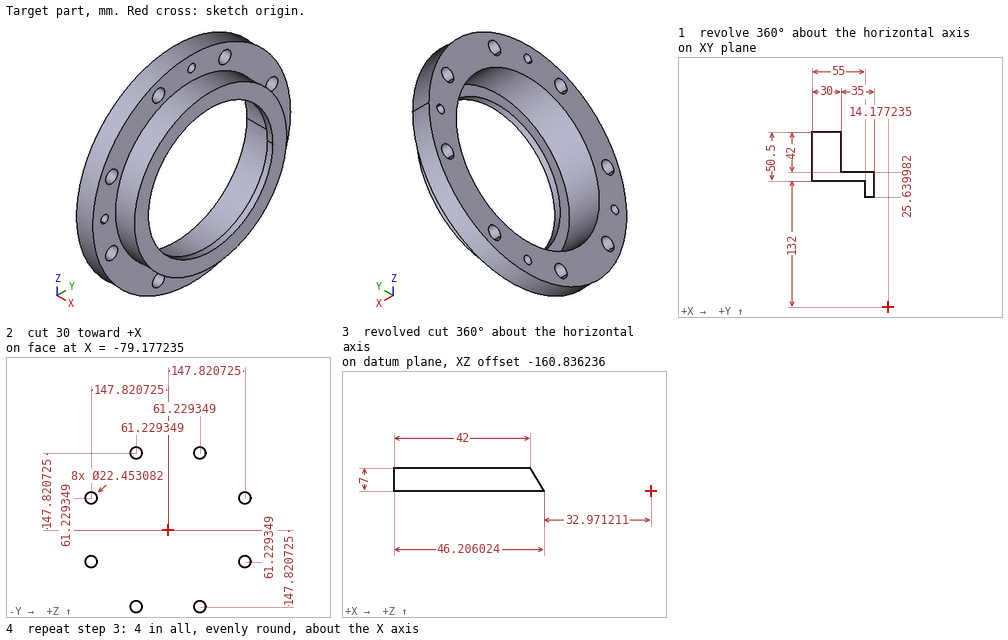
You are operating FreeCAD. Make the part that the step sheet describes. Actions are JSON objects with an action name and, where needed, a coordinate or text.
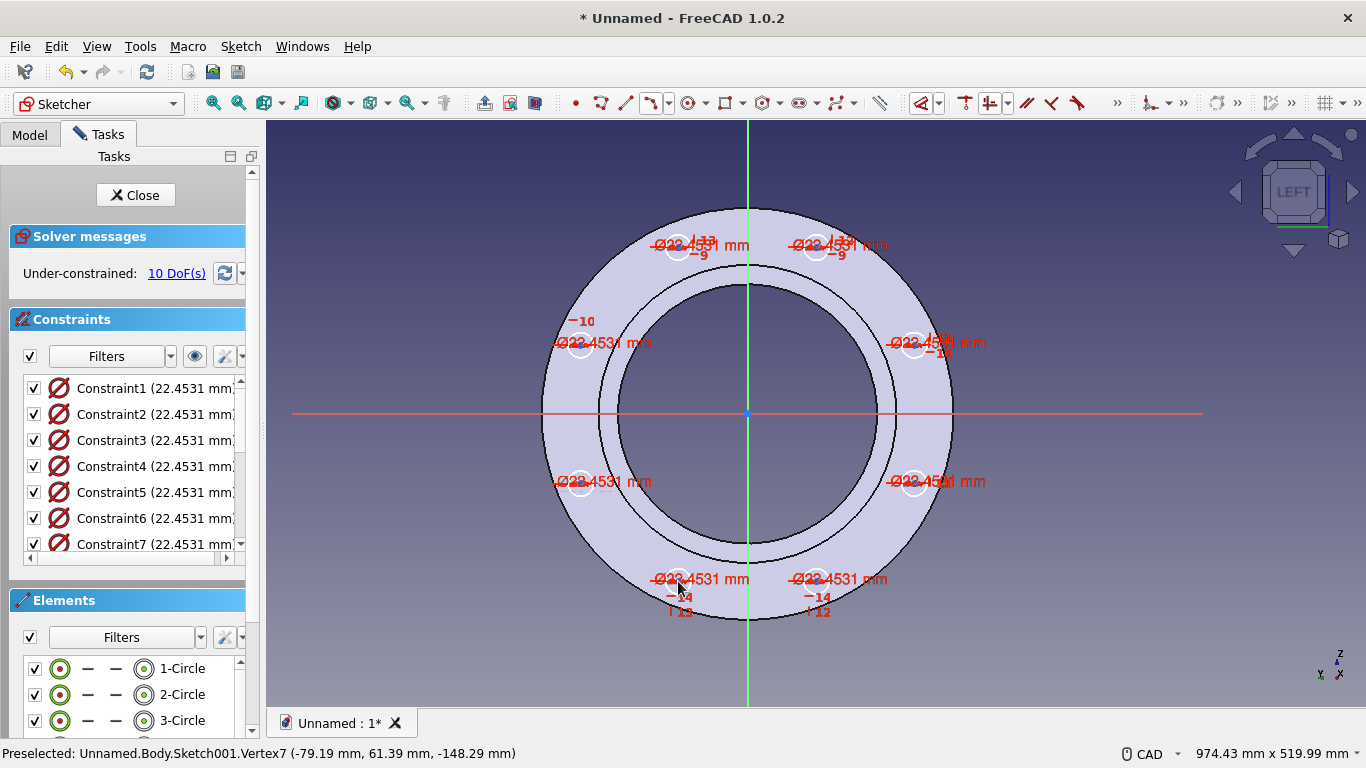
{"action": "left_click", "coordinate": [581, 345]}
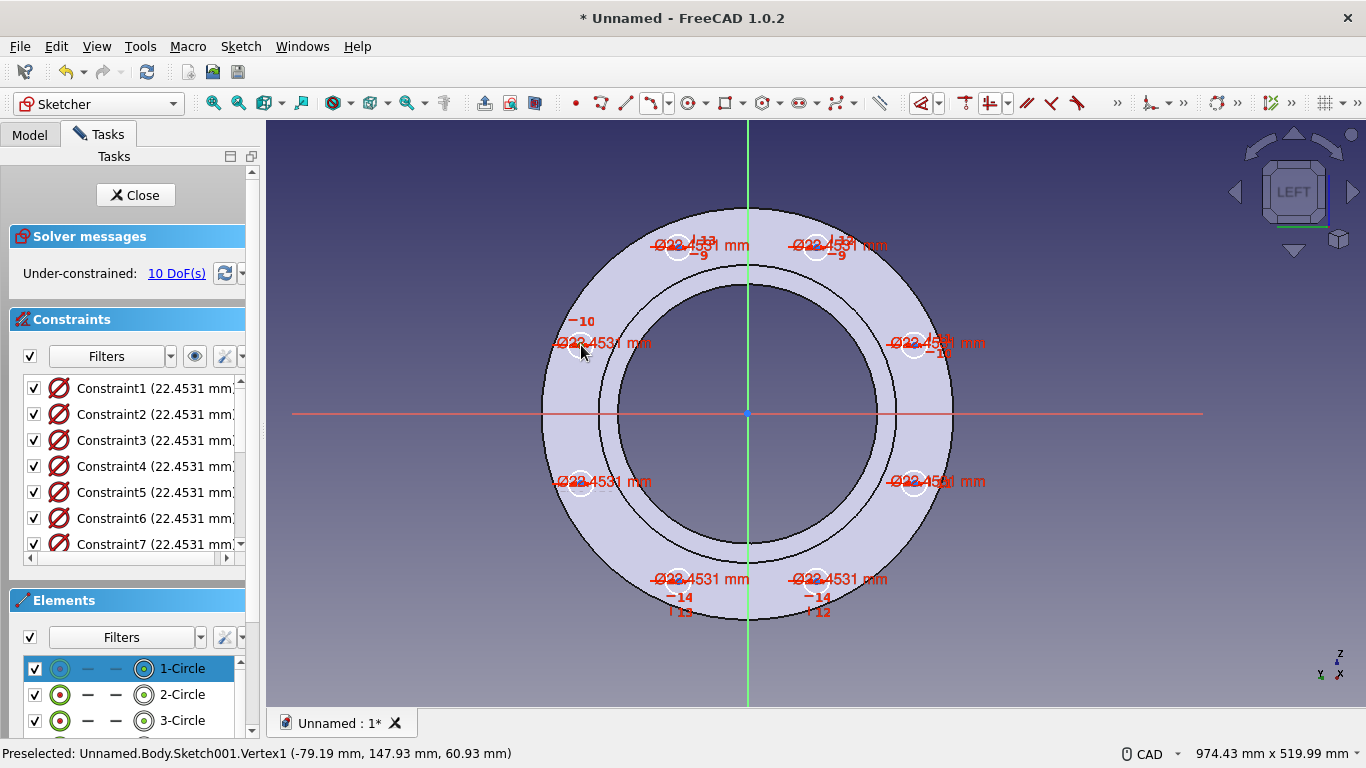
{"action": "left_click", "coordinate": [581, 484]}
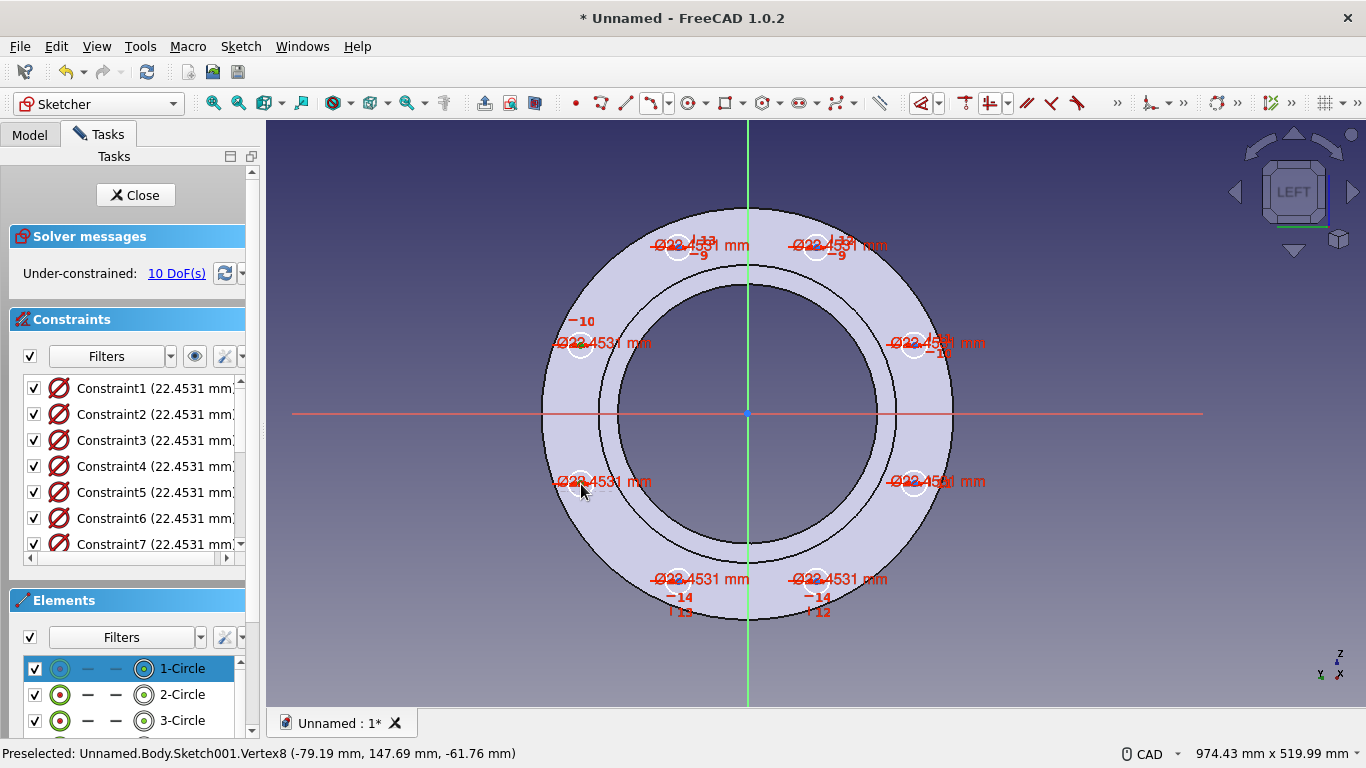
{"action": "left_click", "coordinate": [1008, 104]}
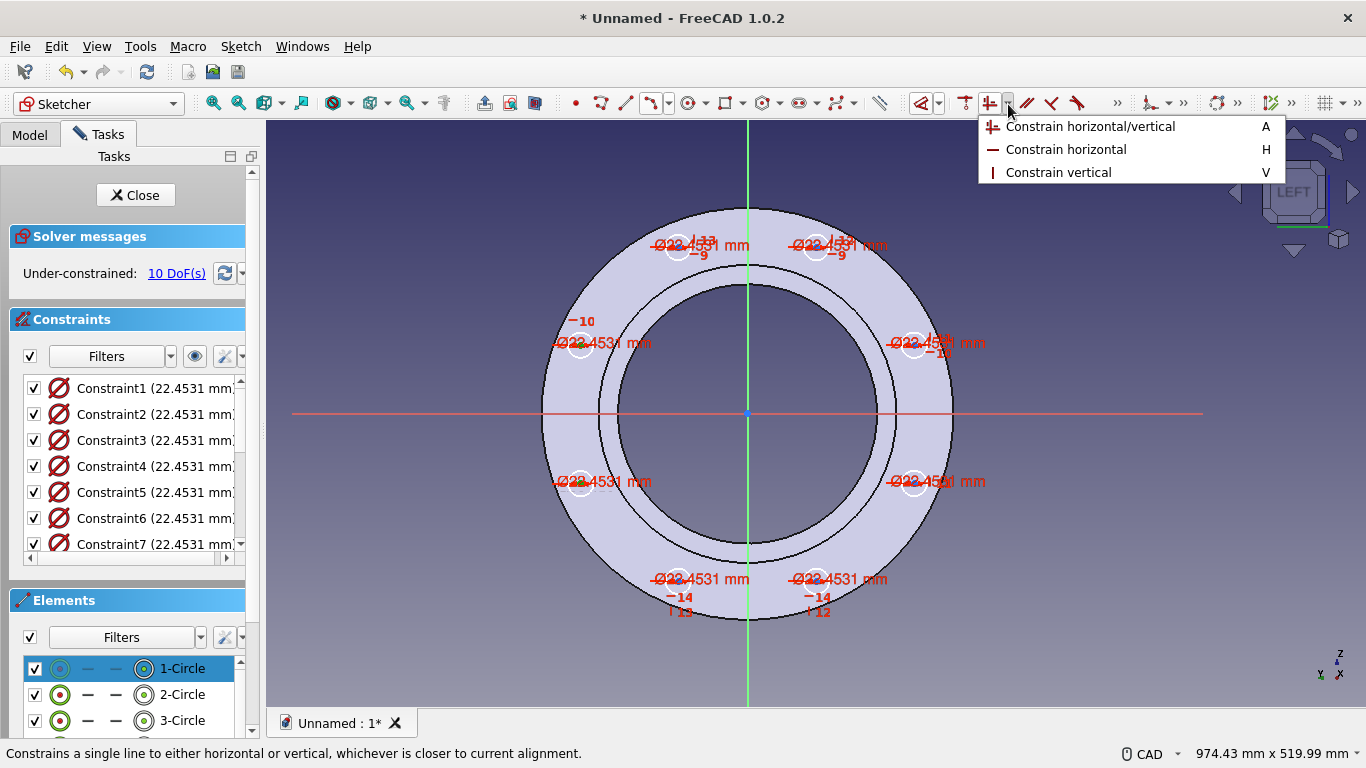
{"action": "left_click", "coordinate": [1132, 172]}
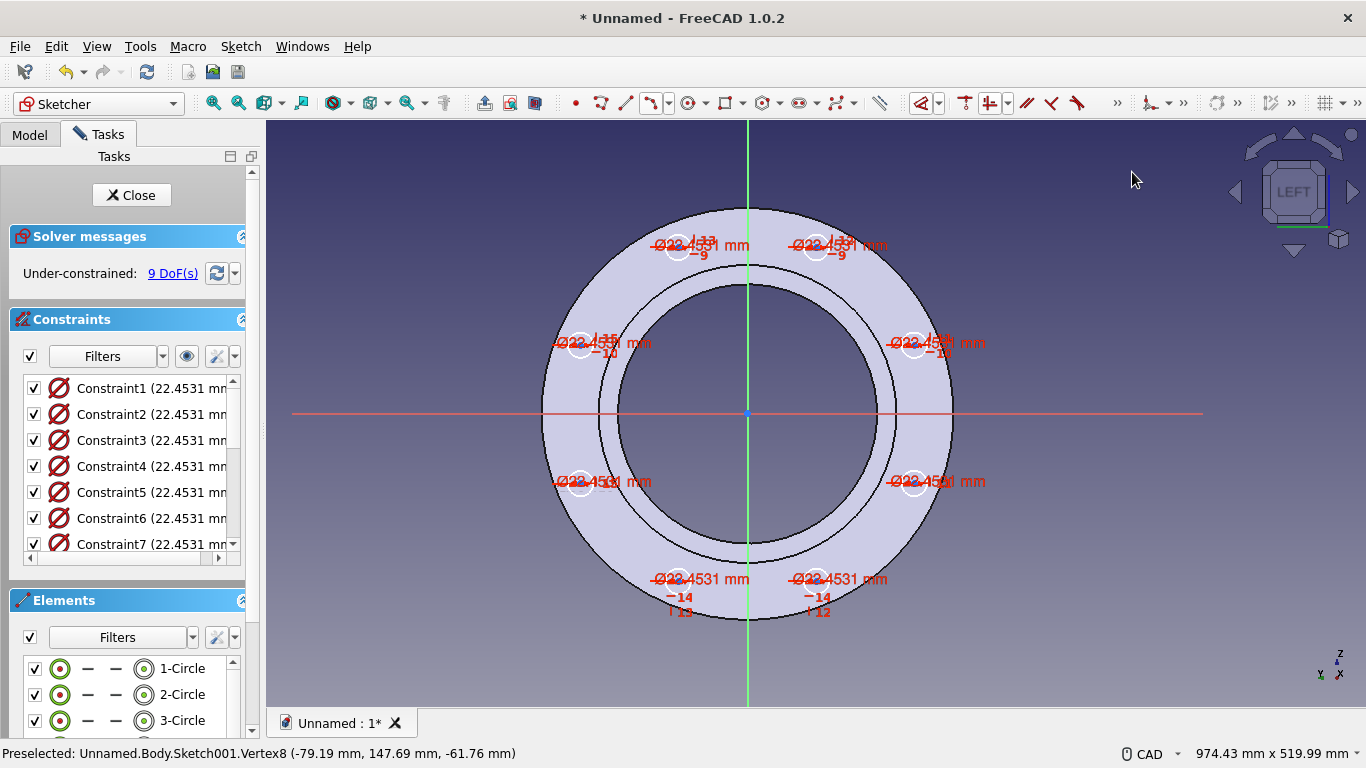
{"action": "left_click", "coordinate": [914, 483]}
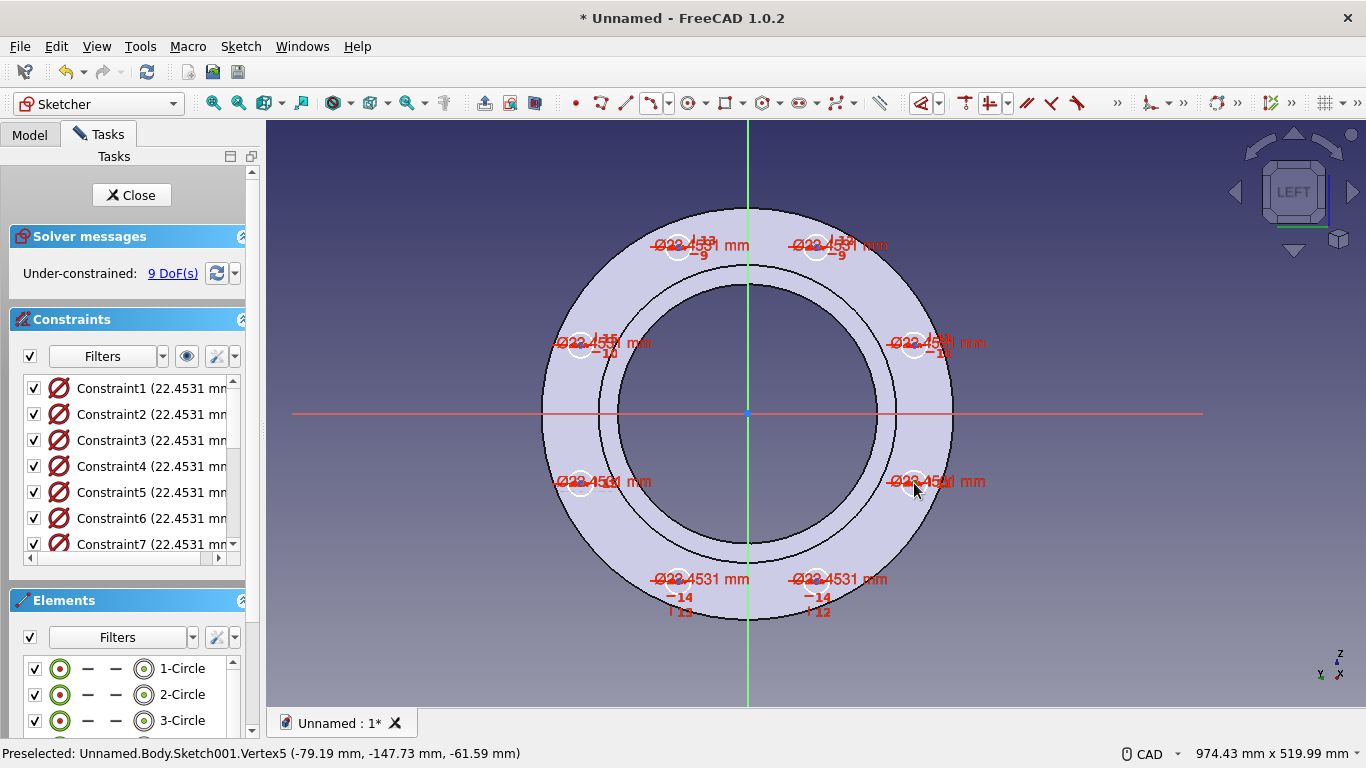
{"action": "left_click", "coordinate": [581, 484]}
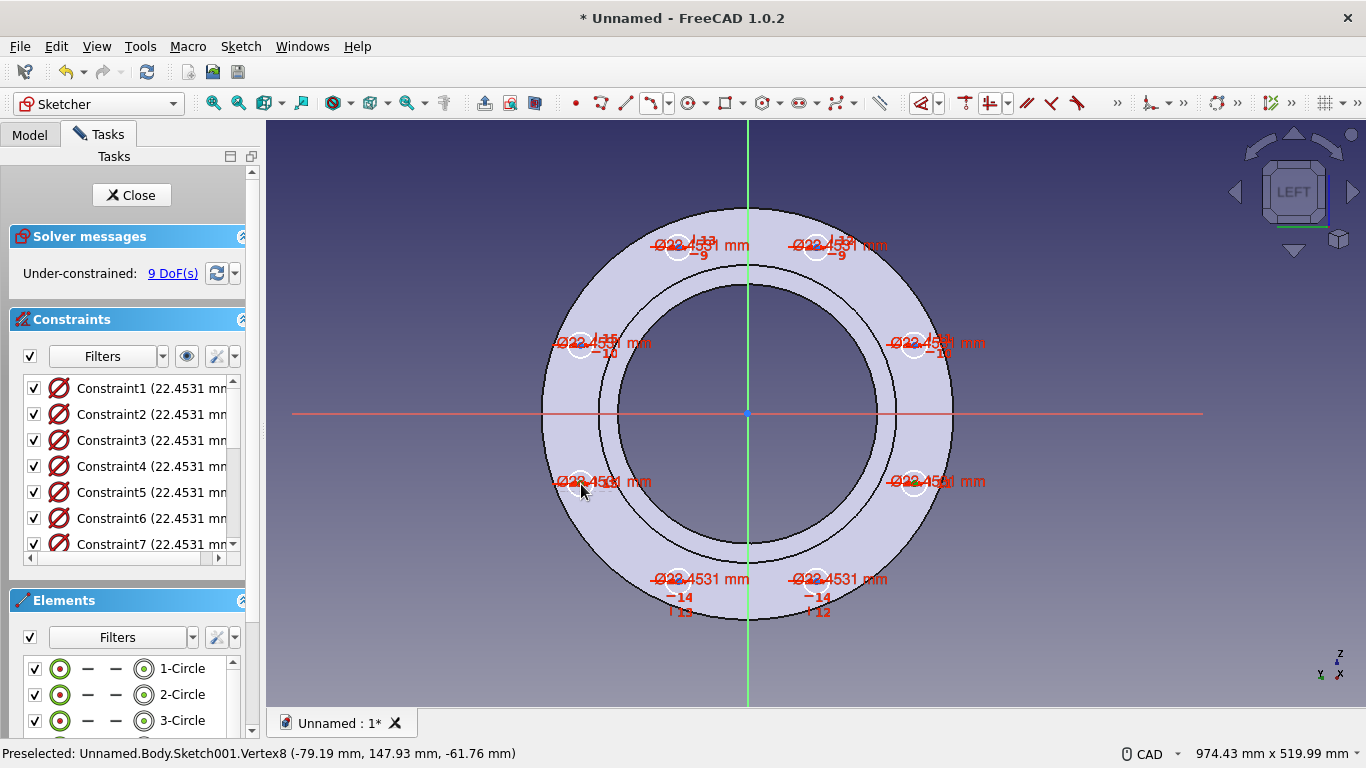
{"action": "left_click", "coordinate": [1008, 104]}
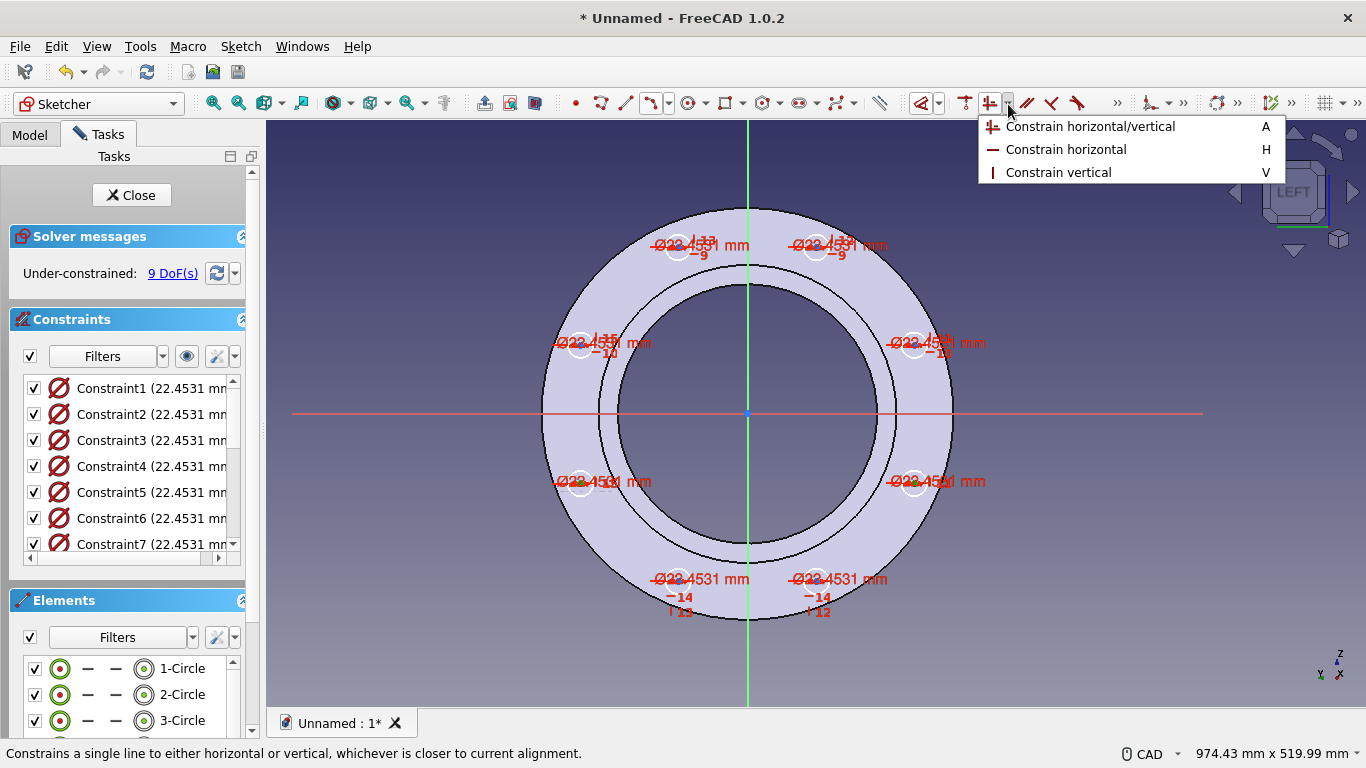
{"action": "left_click", "coordinate": [1132, 150]}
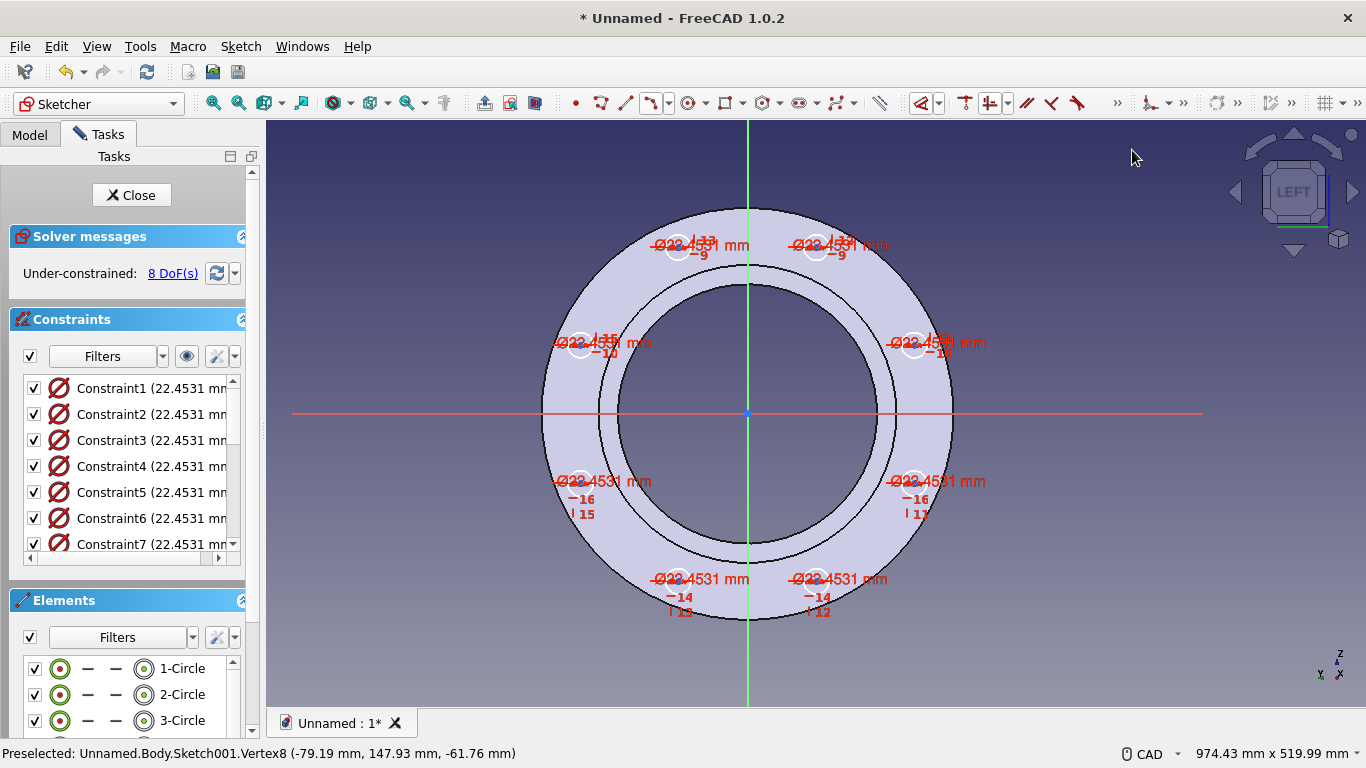
{"action": "left_click", "coordinate": [581, 345]}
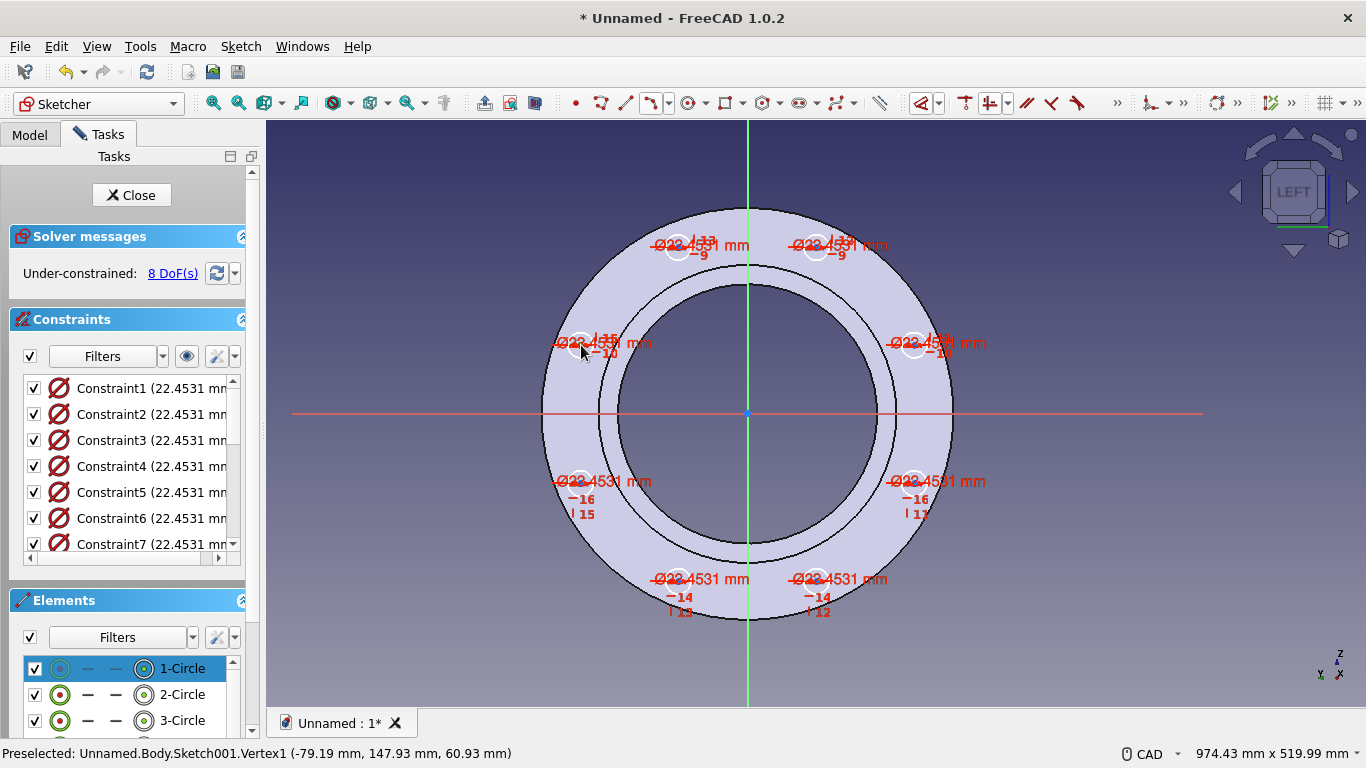
{"action": "key", "text": "i"}